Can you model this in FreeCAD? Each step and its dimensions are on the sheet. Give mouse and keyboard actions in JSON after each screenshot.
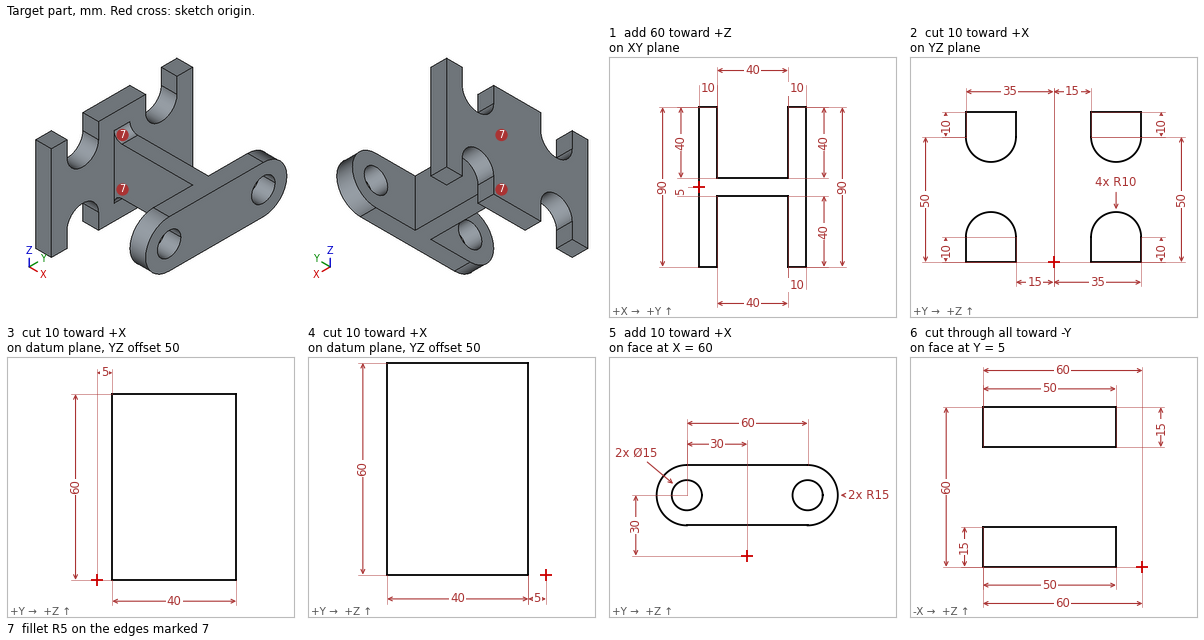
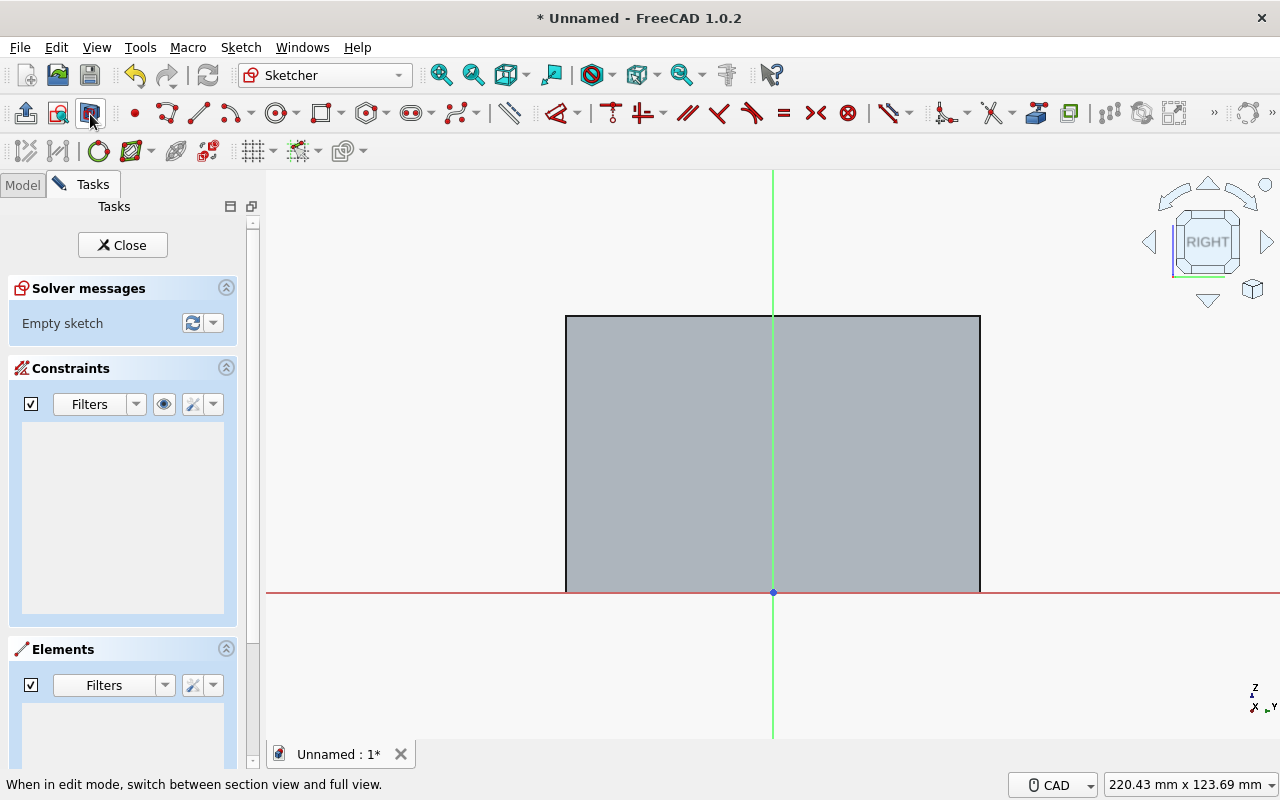
{"action": "left_click", "coordinate": [168, 114]}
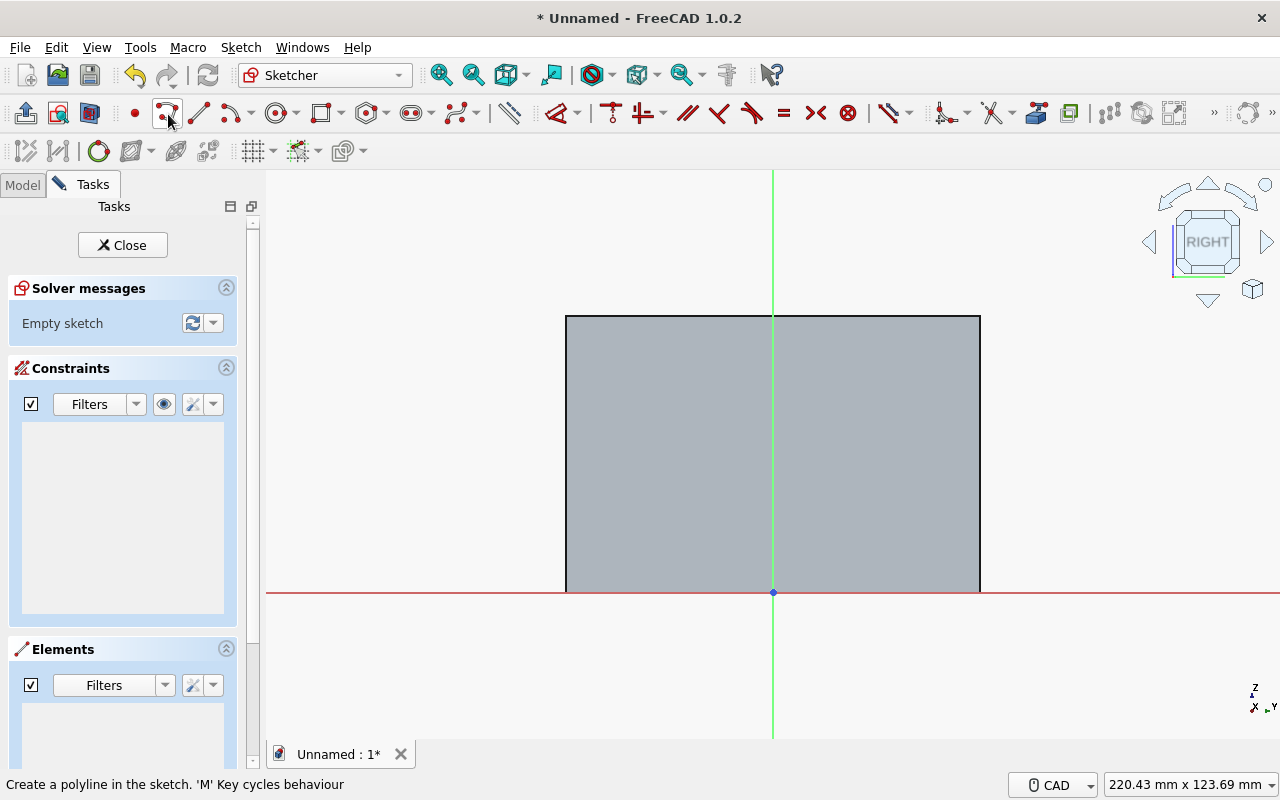
{"action": "left_click", "coordinate": [934, 547]}
{"action": "left_click", "coordinate": [934, 593]}
{"action": "left_click", "coordinate": [842, 584]}
{"action": "left_click", "coordinate": [842, 547]}
{"action": "right_click", "coordinate": [842, 547]}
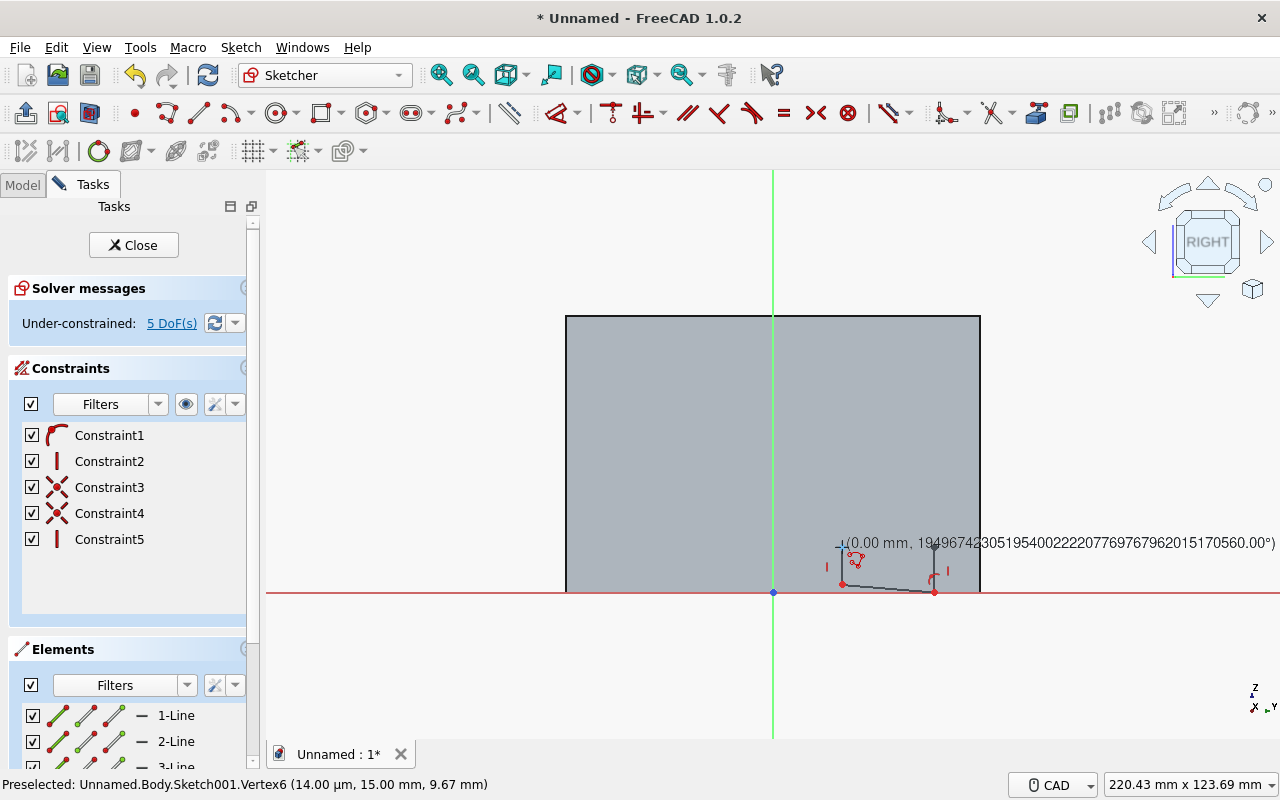
{"action": "left_click", "coordinate": [254, 114]}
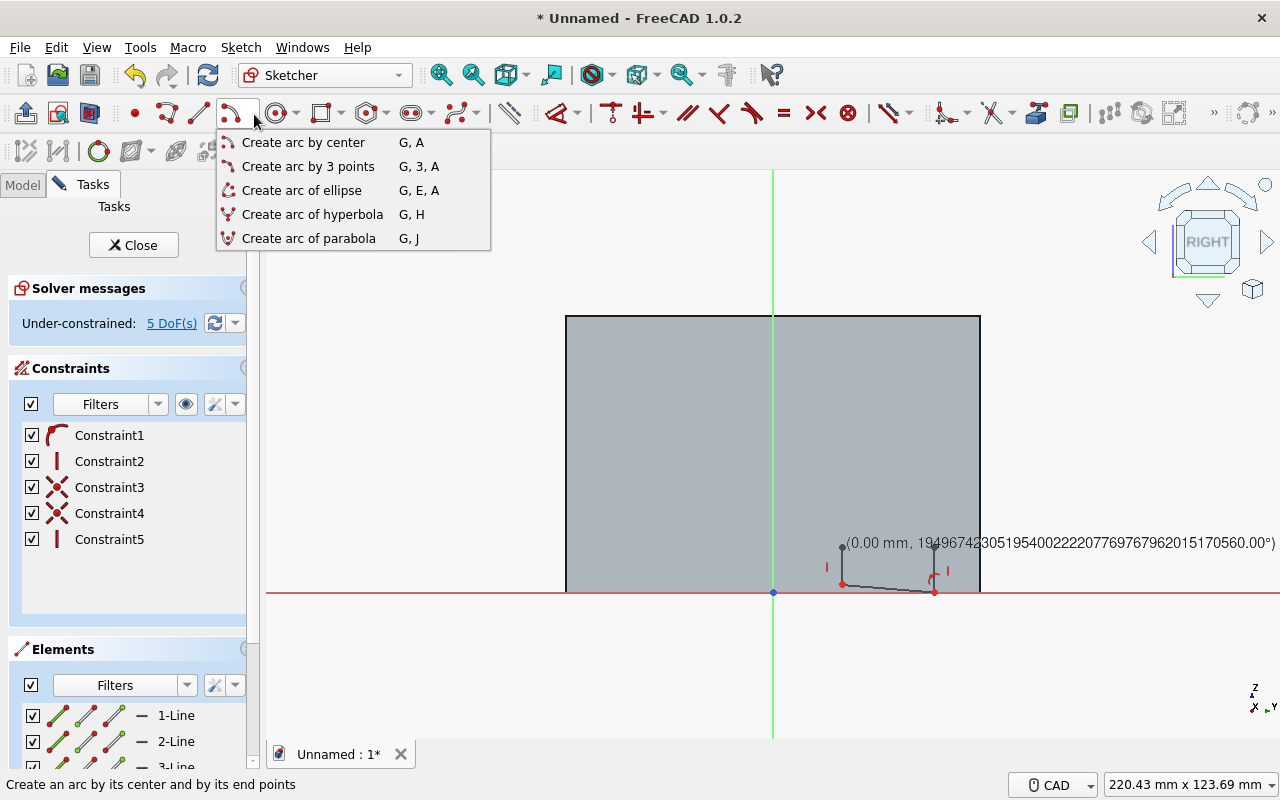
{"action": "left_click", "coordinate": [354, 166]}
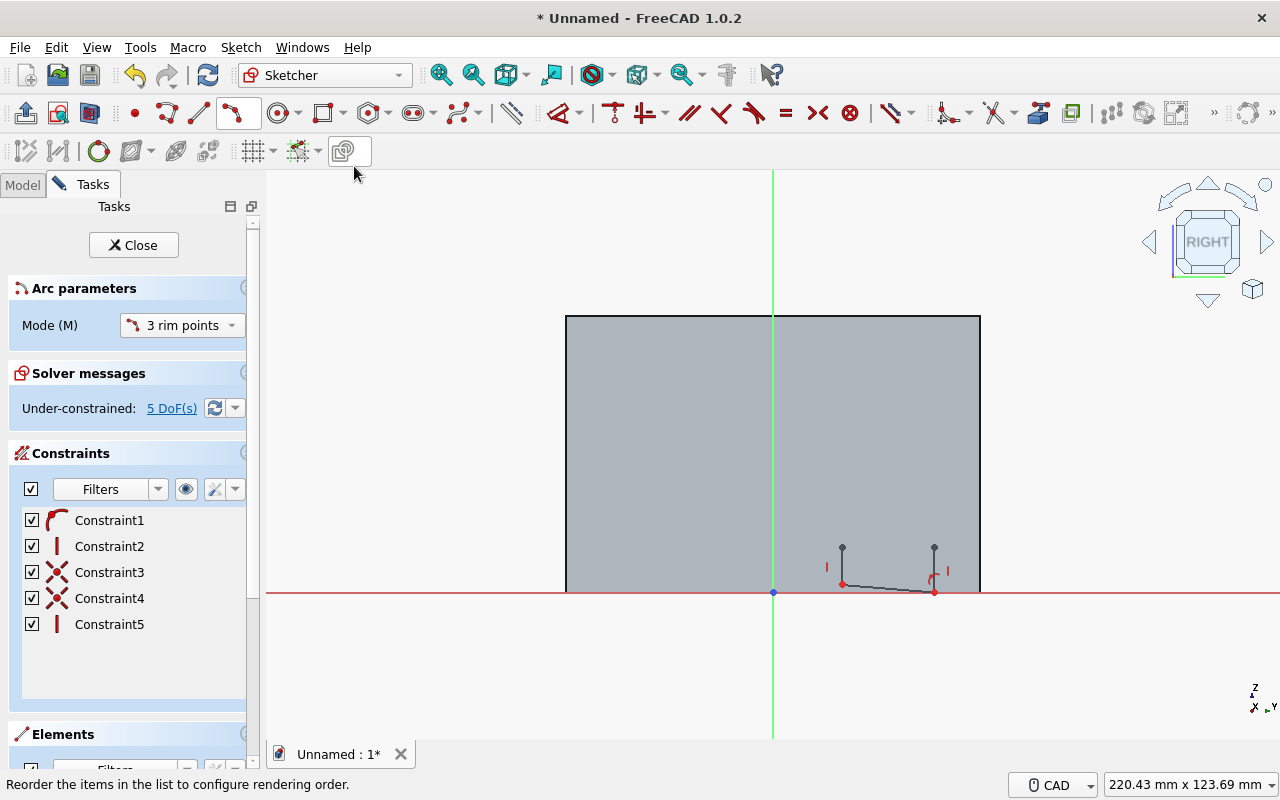
{"action": "left_click", "coordinate": [842, 548]}
{"action": "left_click", "coordinate": [934, 548]}
{"action": "left_click", "coordinate": [888, 501]}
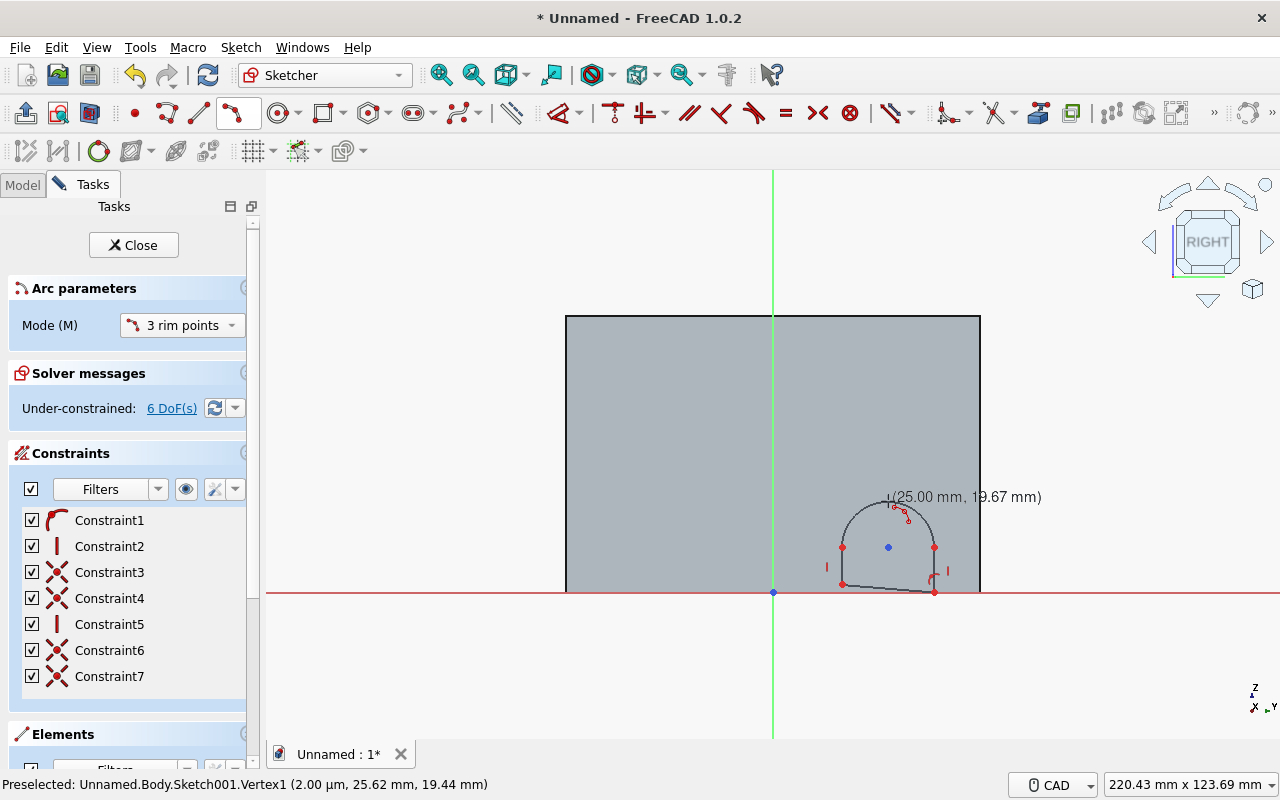
{"action": "left_click", "coordinate": [168, 114]}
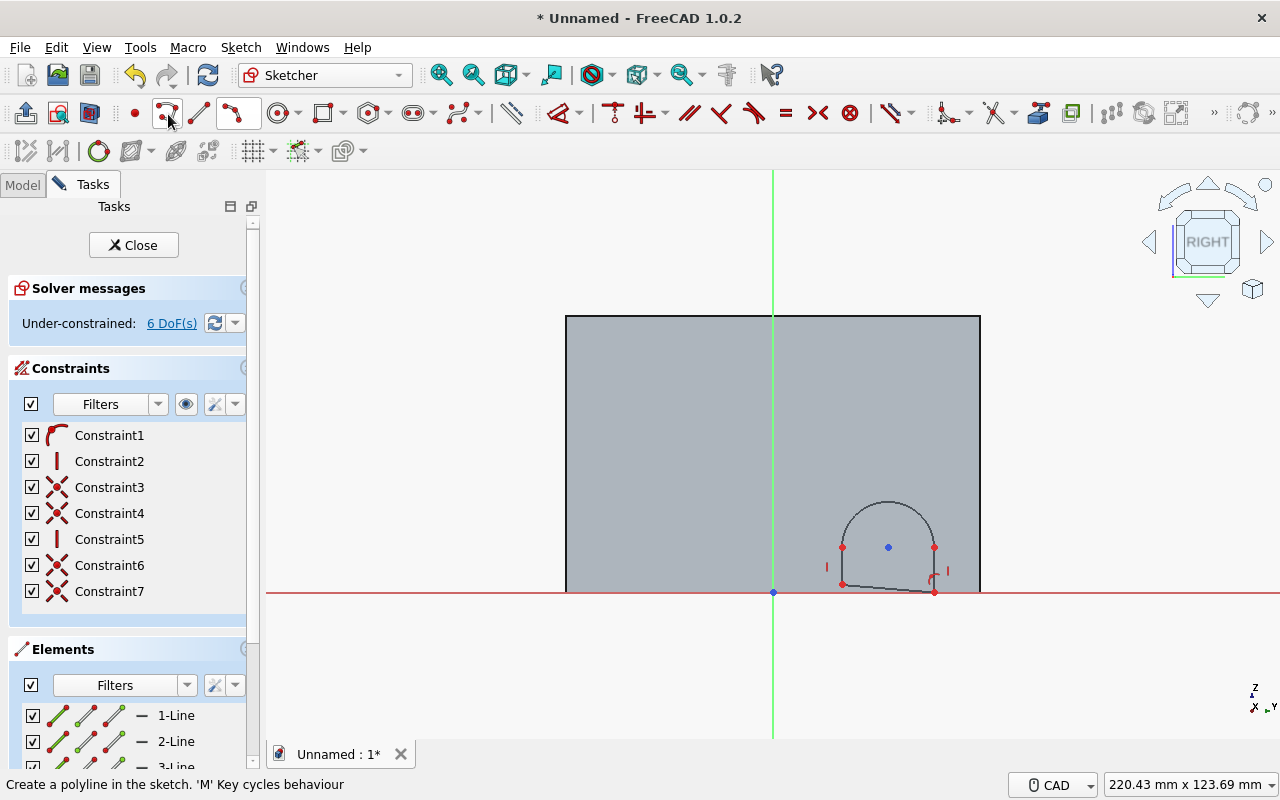
{"action": "left_click", "coordinate": [842, 362]}
{"action": "left_click", "coordinate": [842, 316]}
{"action": "left_click", "coordinate": [934, 316]}
{"action": "left_click", "coordinate": [934, 362]}
{"action": "right_click", "coordinate": [934, 362]}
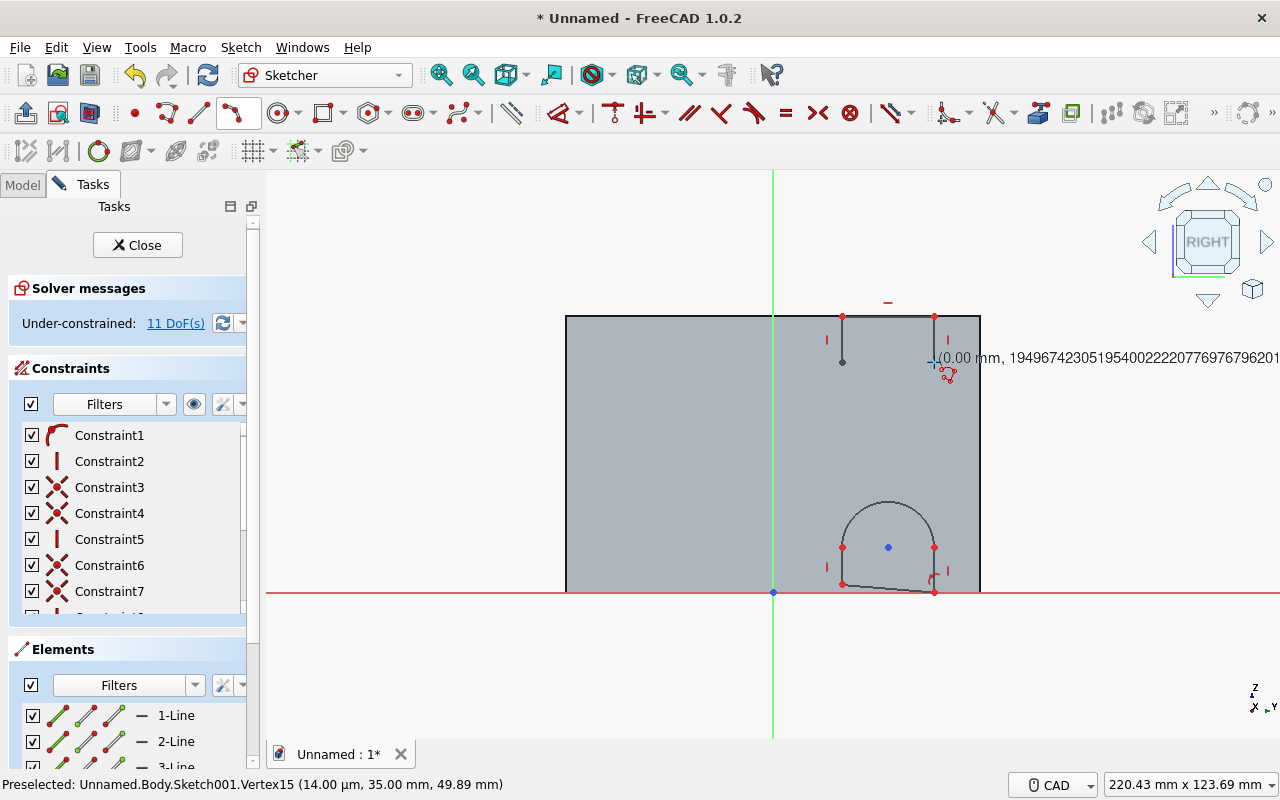
{"action": "left_click", "coordinate": [232, 114]}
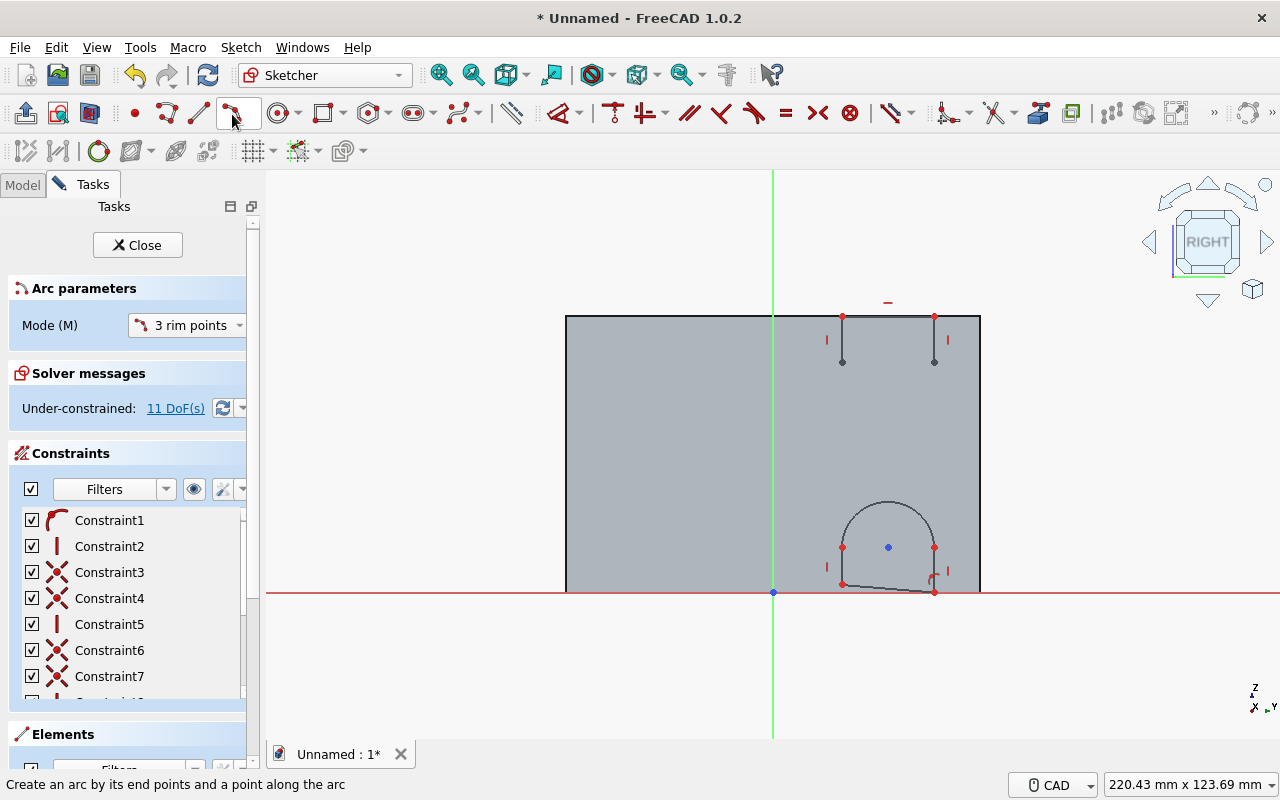
{"action": "left_click", "coordinate": [934, 363]}
{"action": "left_click", "coordinate": [842, 363]}
{"action": "left_click", "coordinate": [888, 408]}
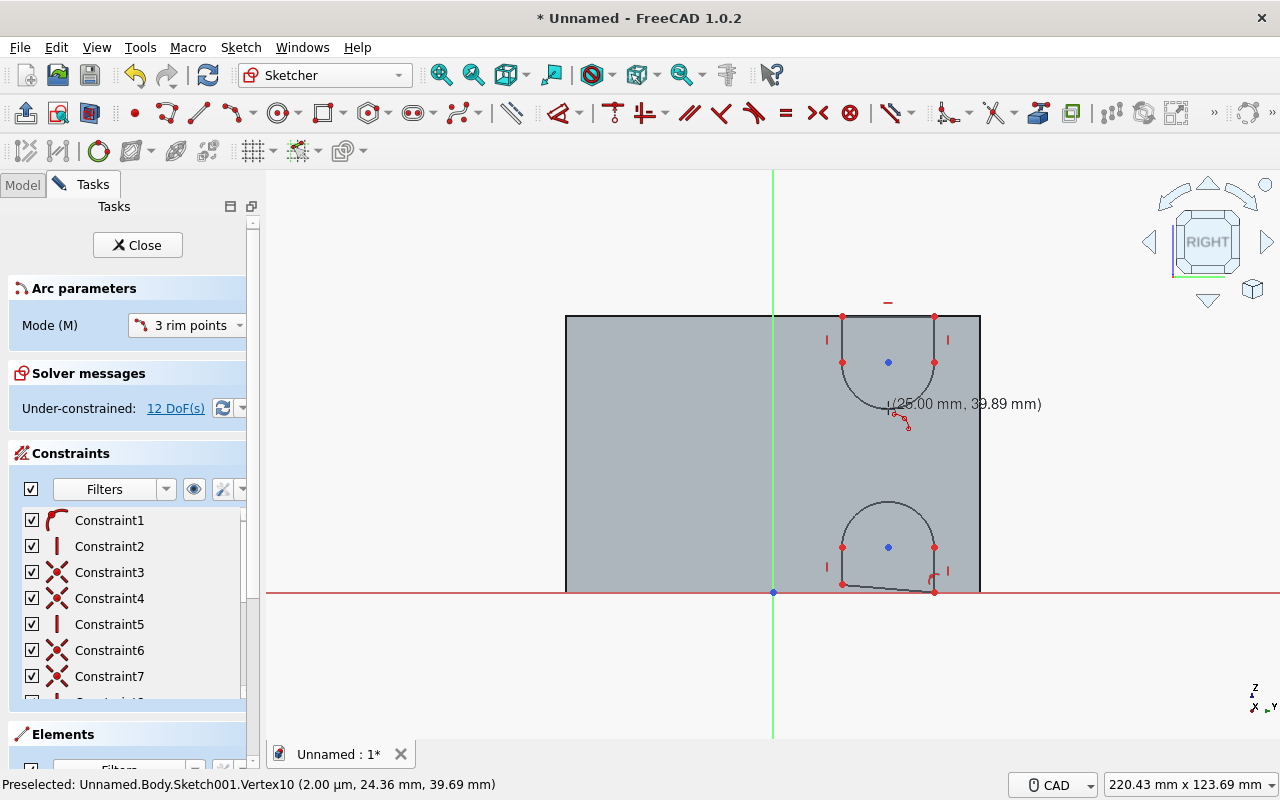
{"action": "left_click", "coordinate": [168, 114]}